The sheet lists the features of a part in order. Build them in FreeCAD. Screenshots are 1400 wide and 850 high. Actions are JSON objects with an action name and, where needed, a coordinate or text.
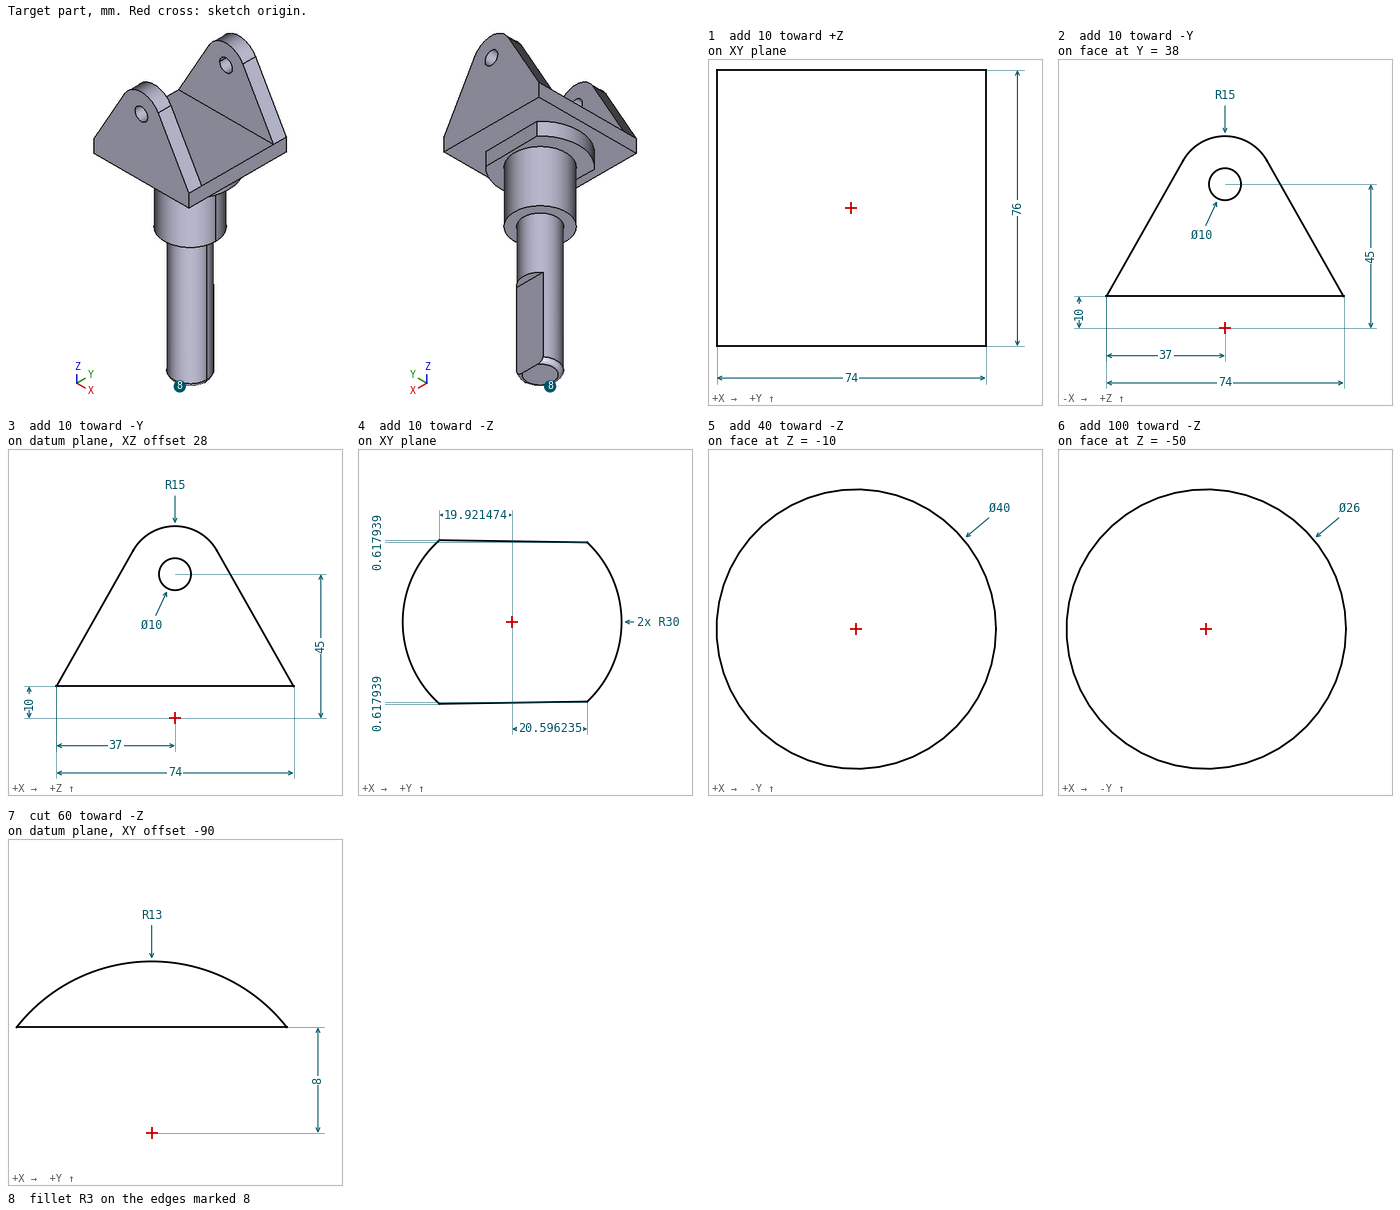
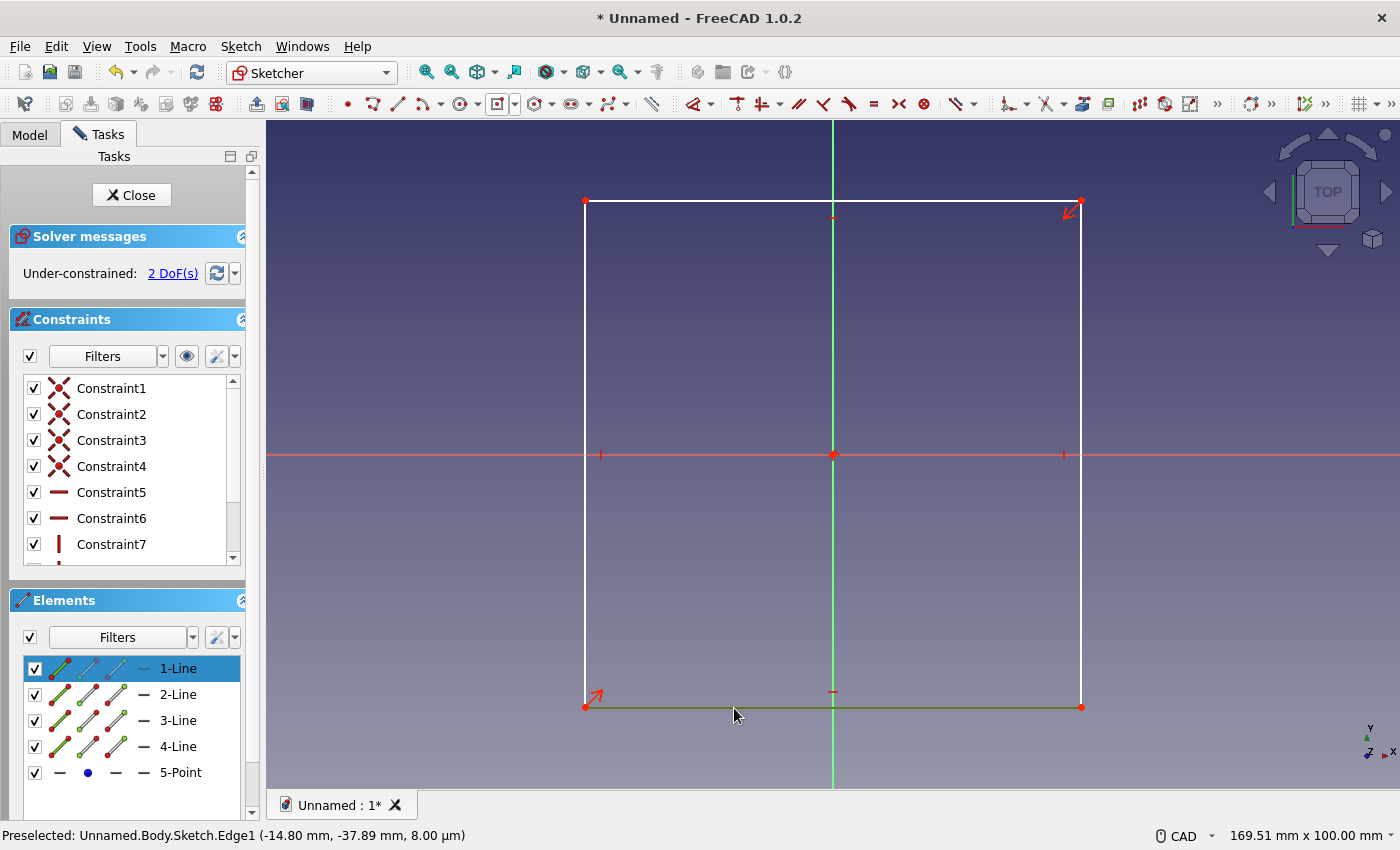
{"action": "key", "text": "l"}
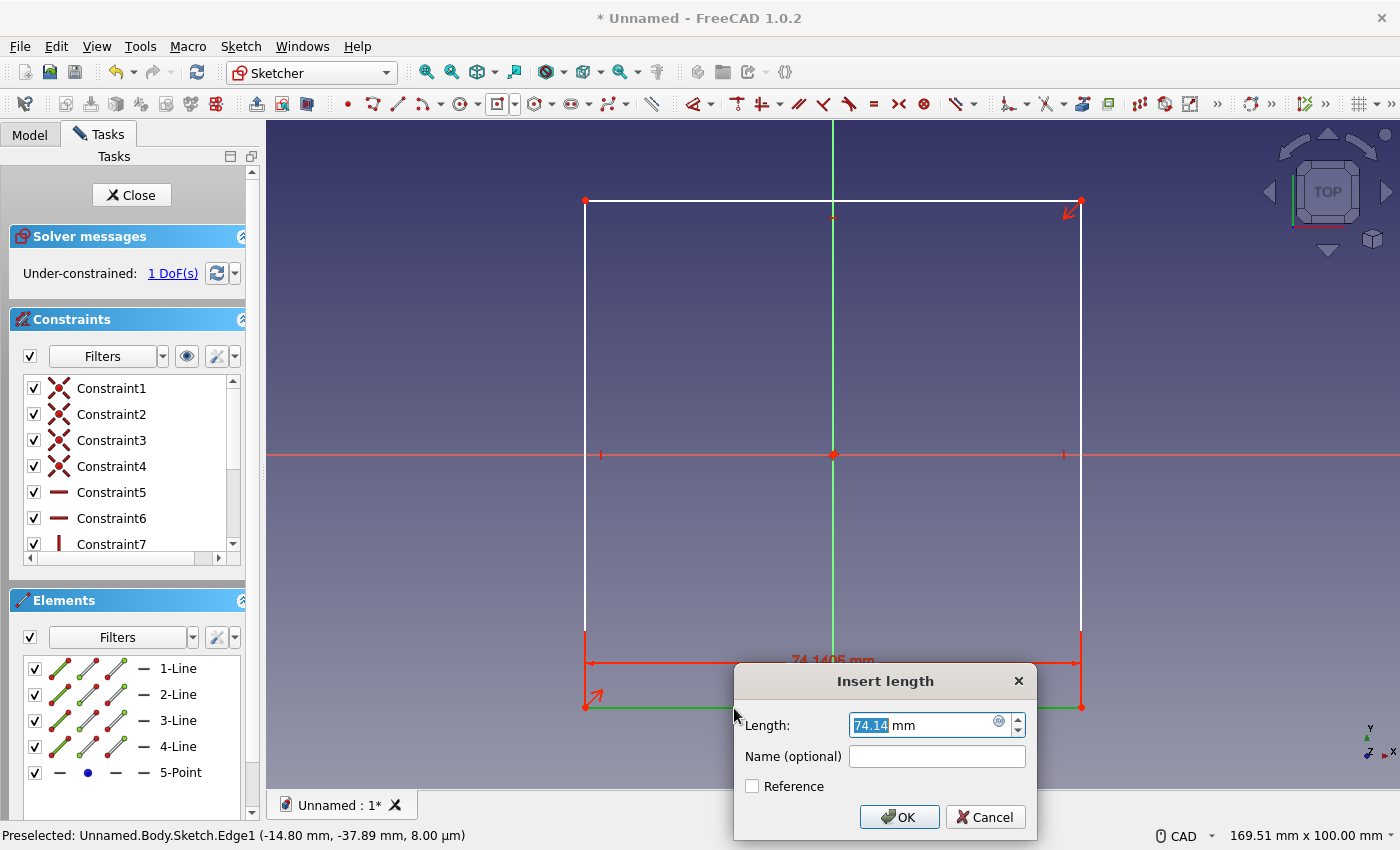
{"action": "type", "text": "74"}
{"action": "key", "text": "Return"}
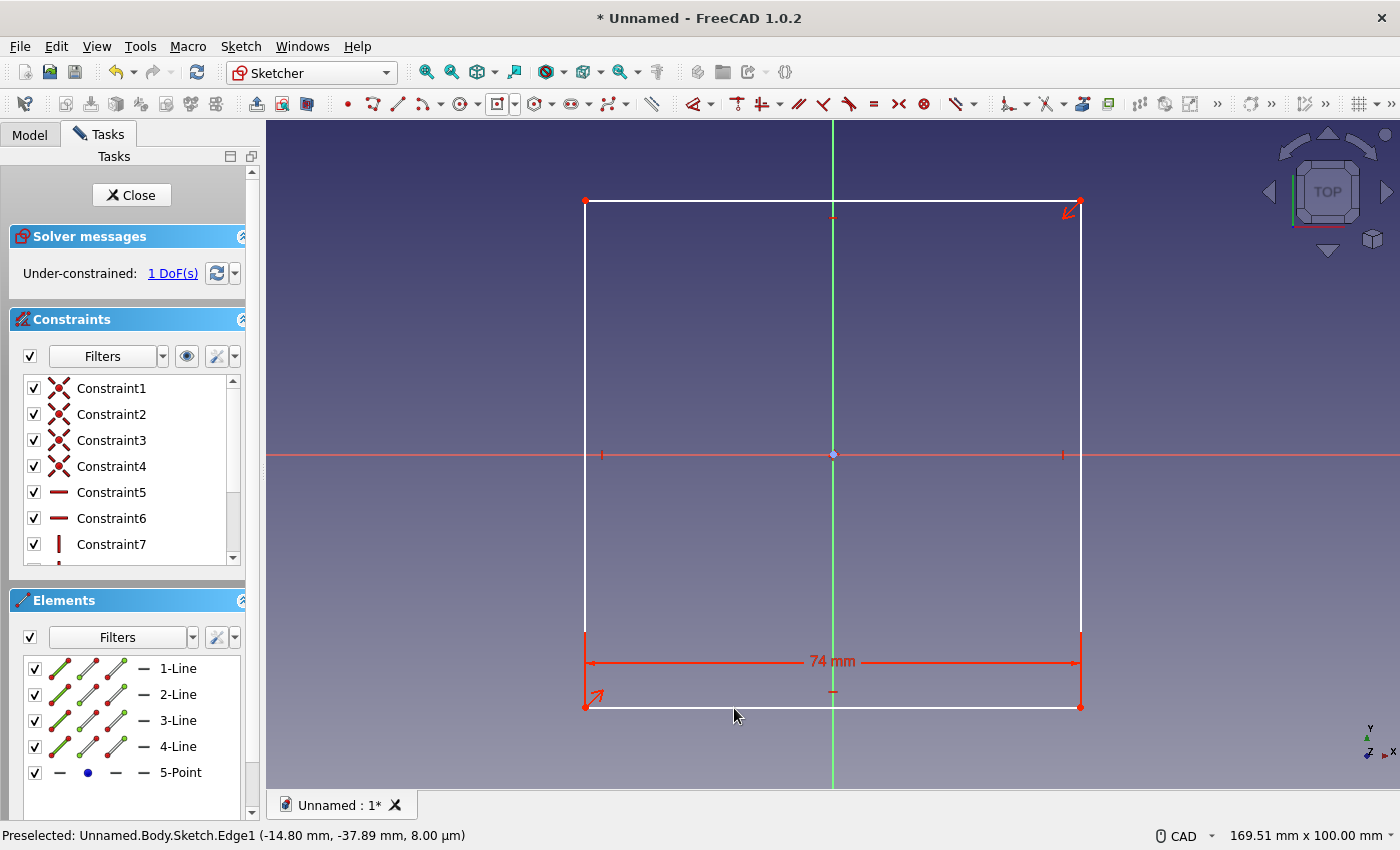
{"action": "left_click", "coordinate": [1081, 556]}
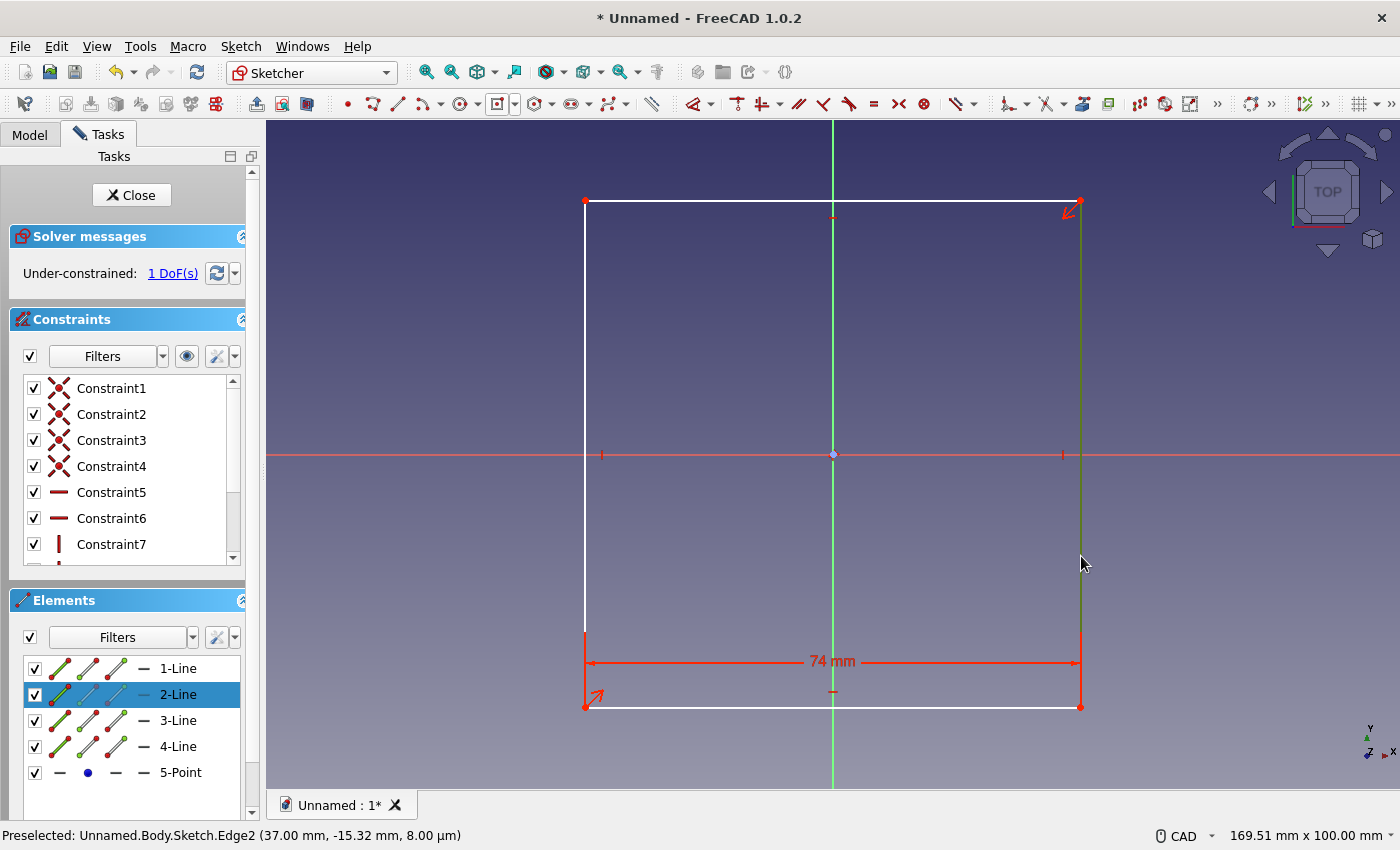
{"action": "left_click", "coordinate": [710, 104]}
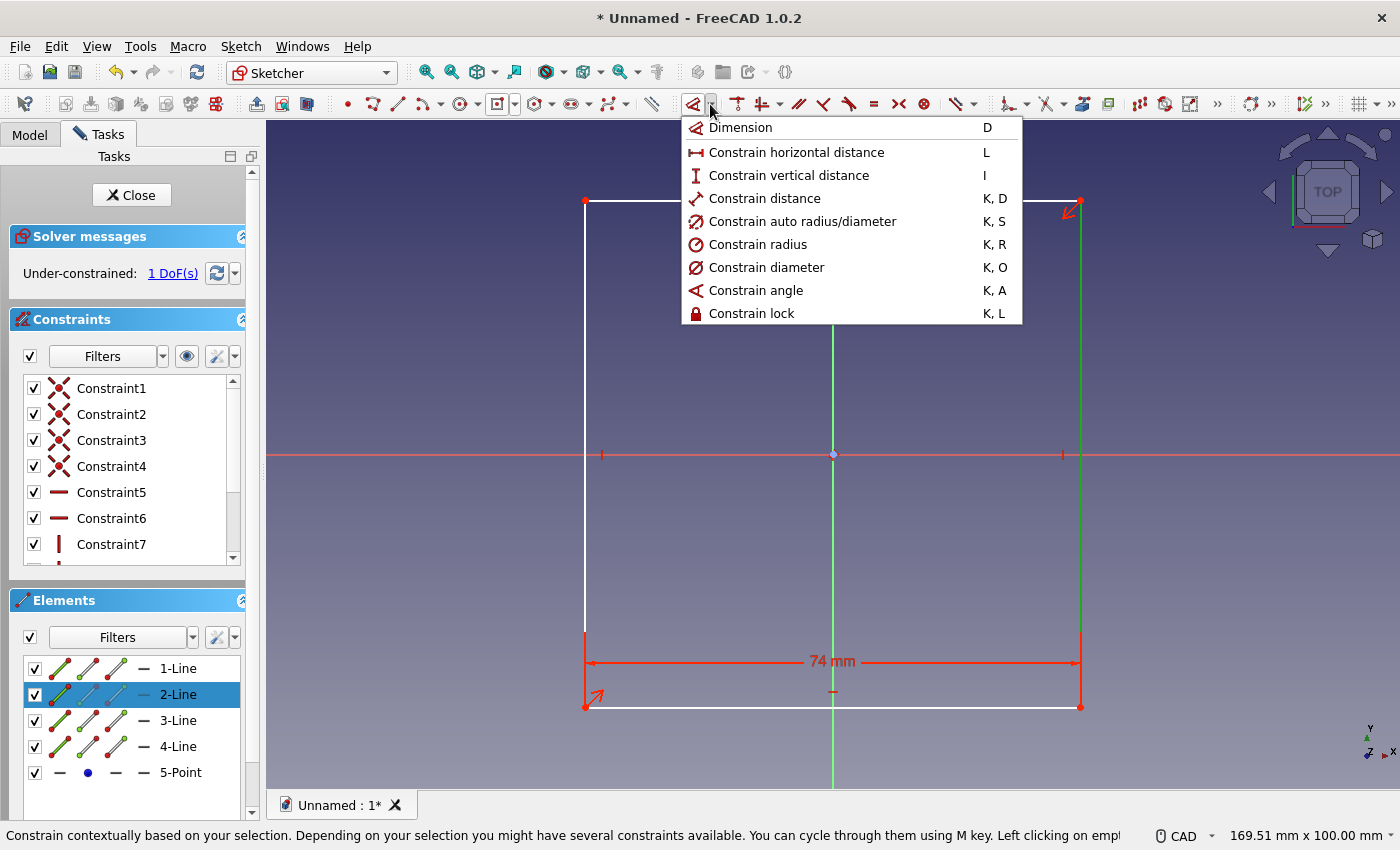
{"action": "left_click", "coordinate": [852, 176]}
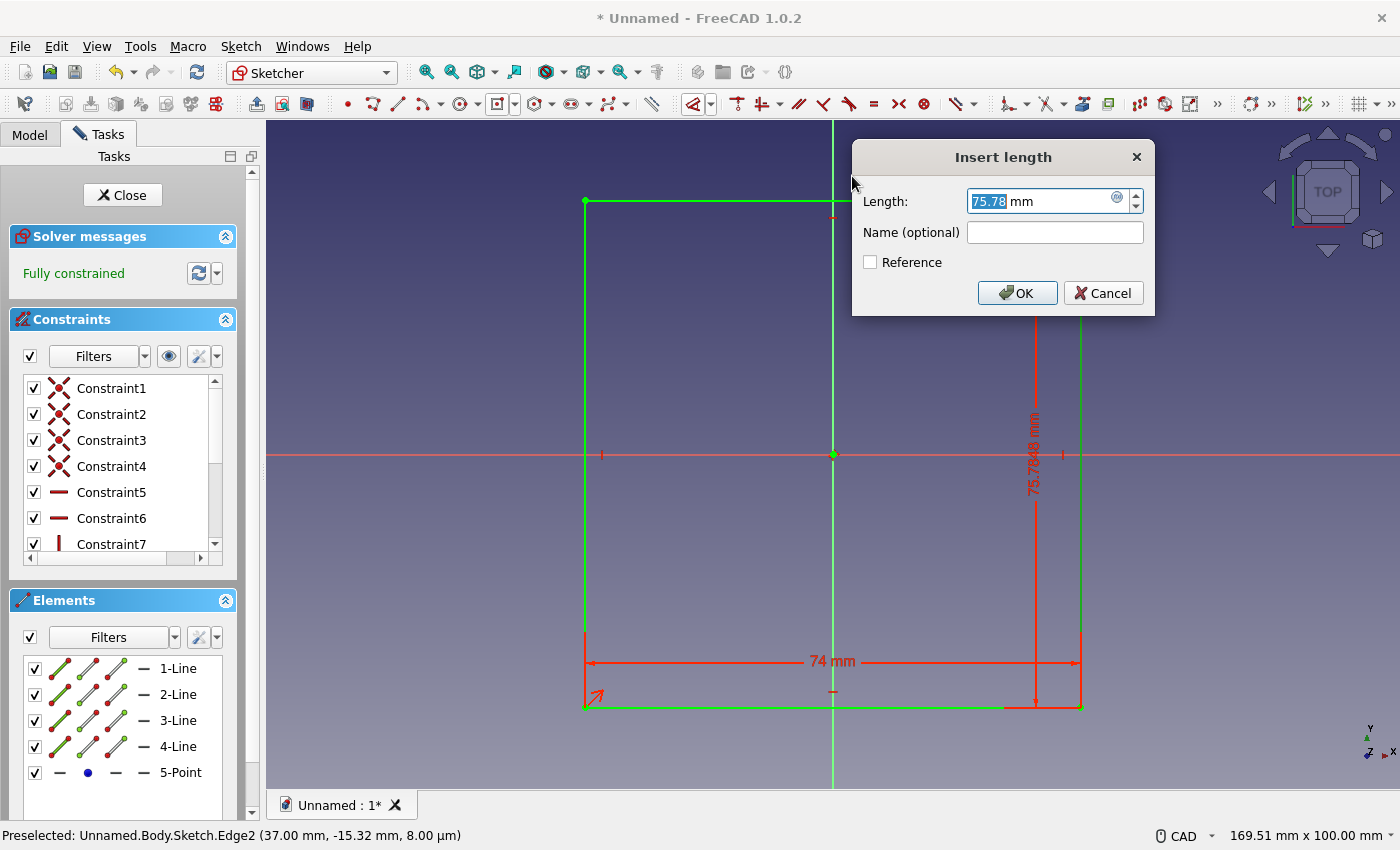
{"action": "type", "text": "76"}
{"action": "key", "text": "Return"}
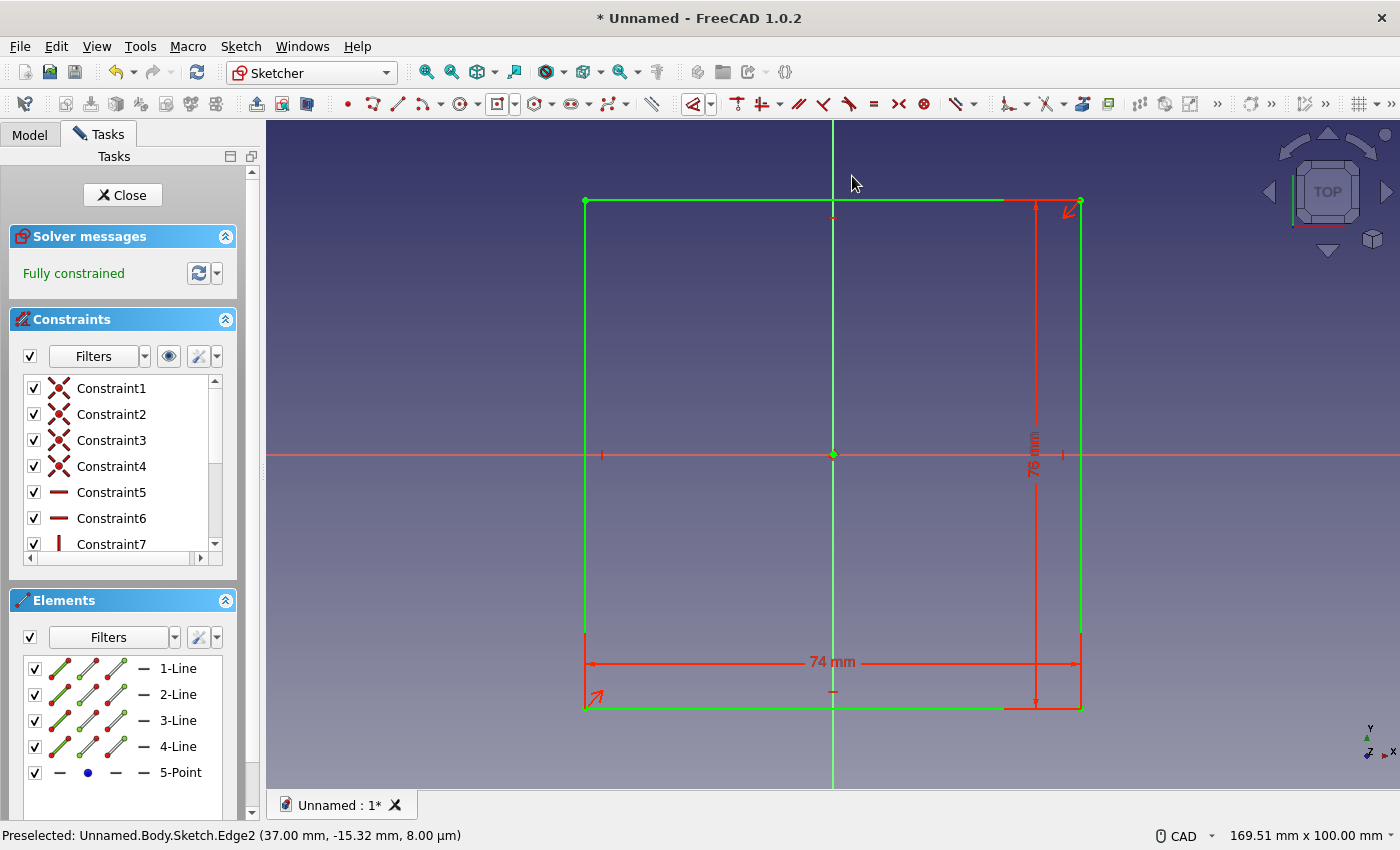
{"action": "left_click", "coordinate": [123, 195]}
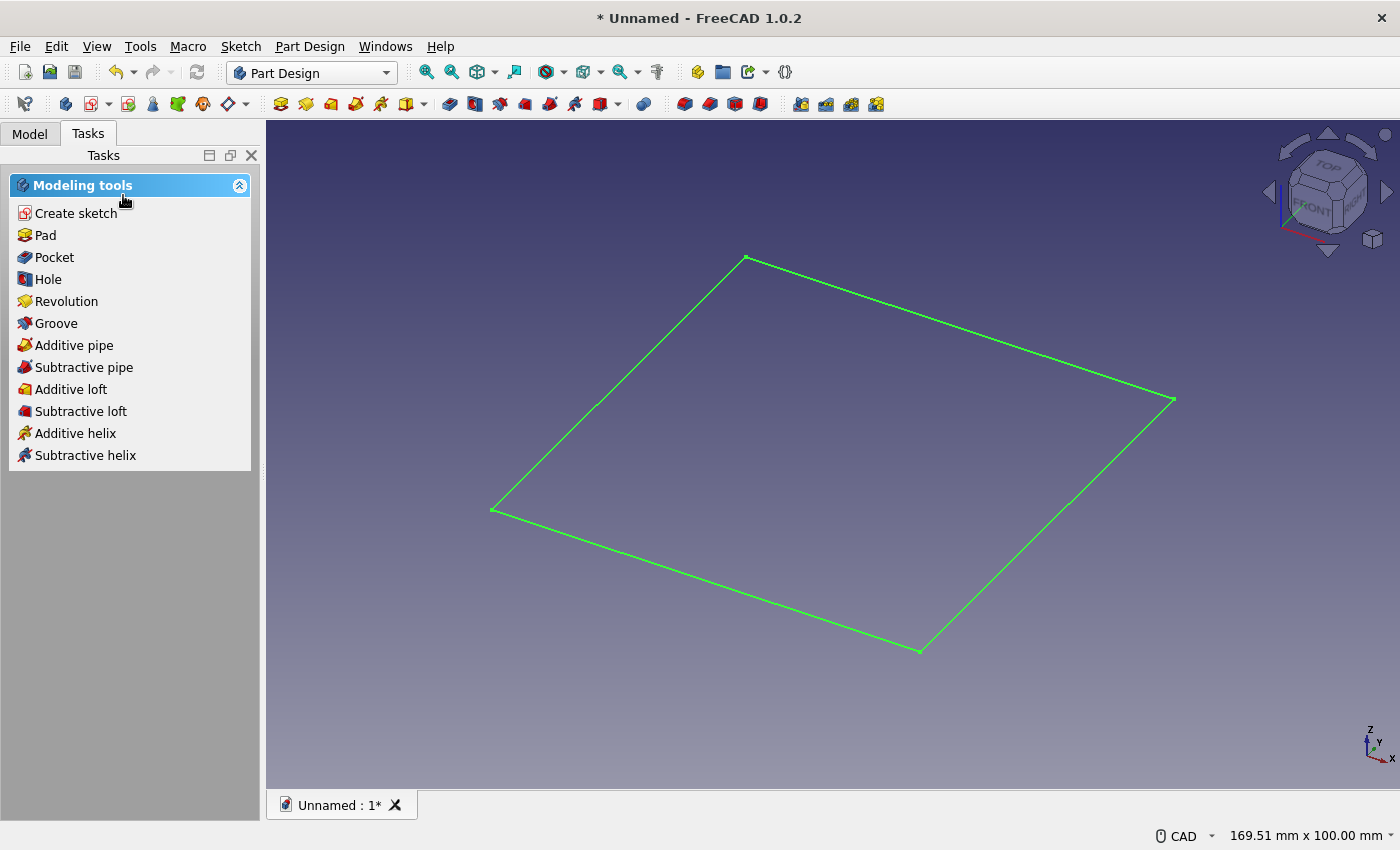
{"action": "left_click", "coordinate": [281, 104]}